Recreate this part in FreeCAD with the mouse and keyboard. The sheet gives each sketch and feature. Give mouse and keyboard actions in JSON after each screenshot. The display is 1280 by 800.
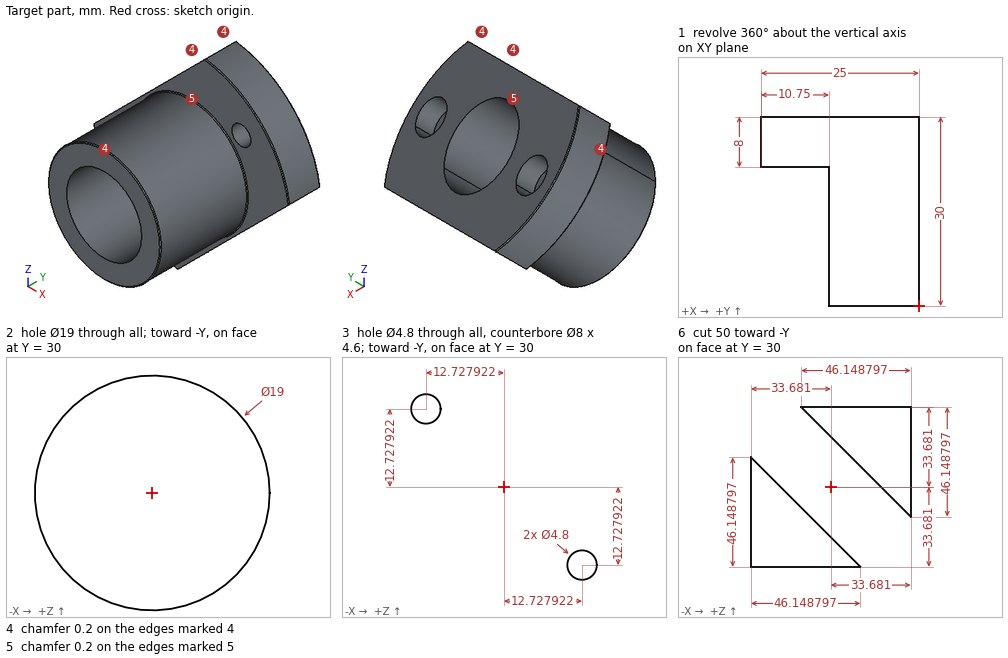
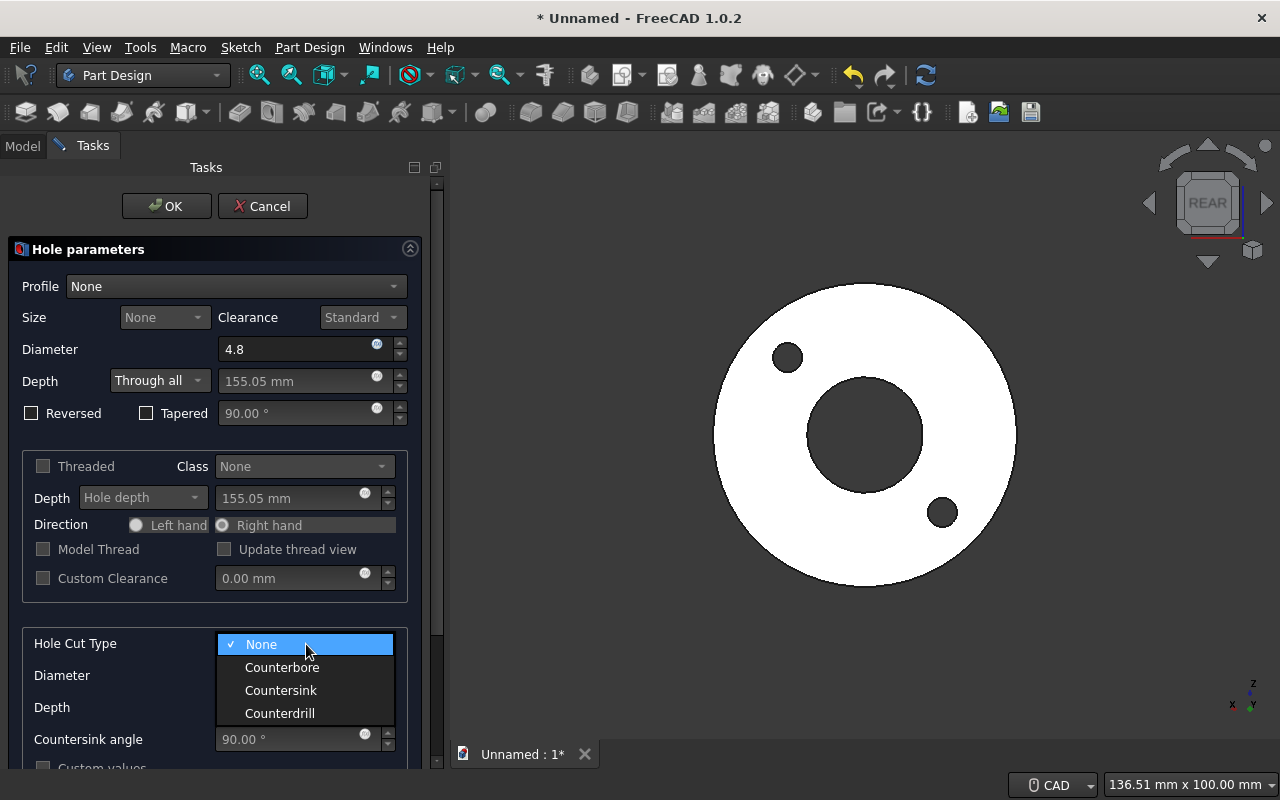
{"action": "left_click", "coordinate": [304, 668]}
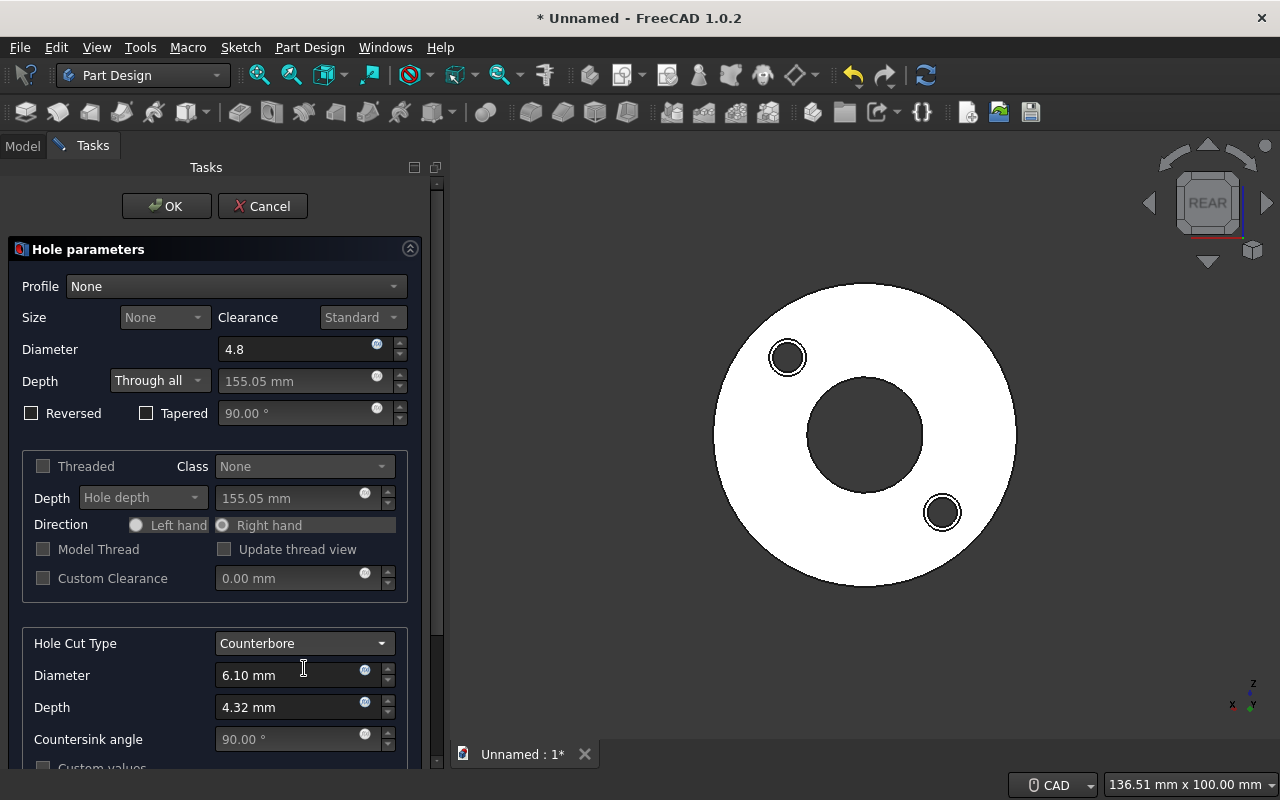
{"action": "triple_click", "coordinate": [298, 675]}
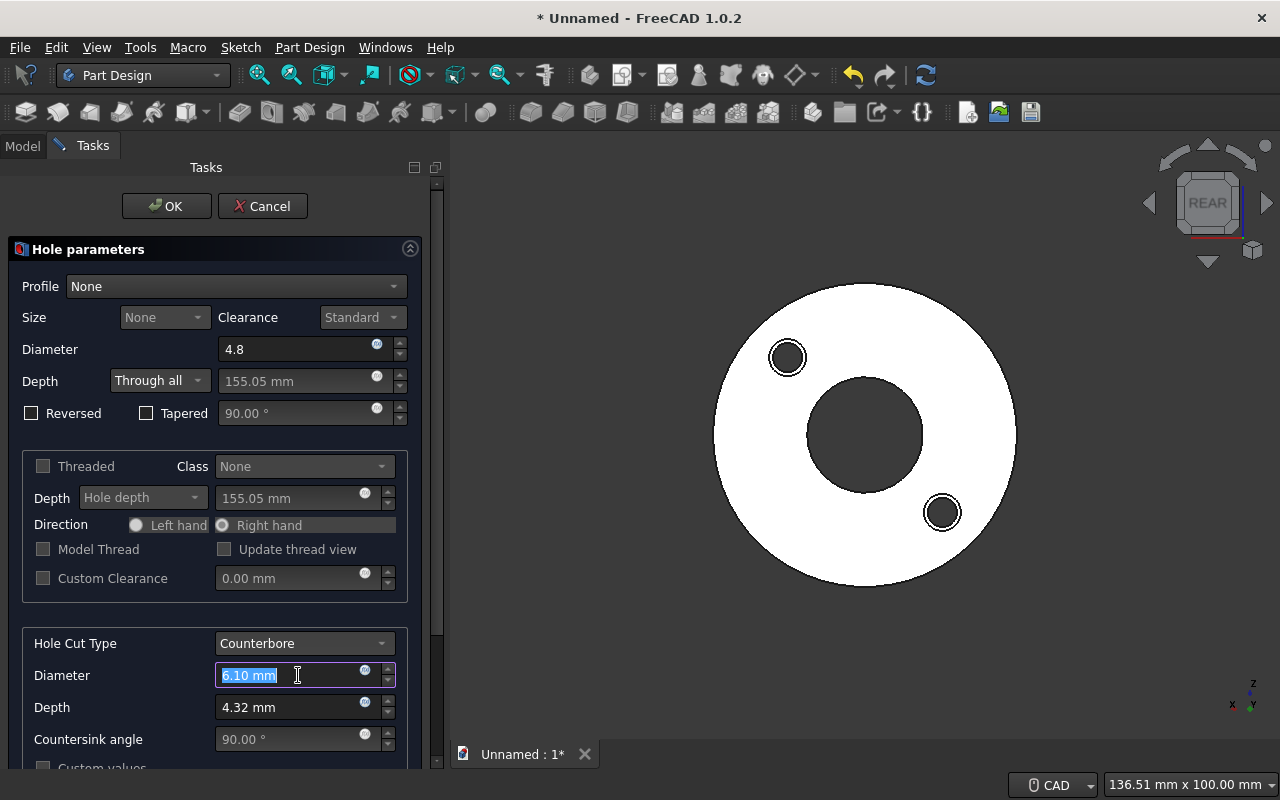
{"action": "type", "text": "8"}
{"action": "key", "text": "Tab"}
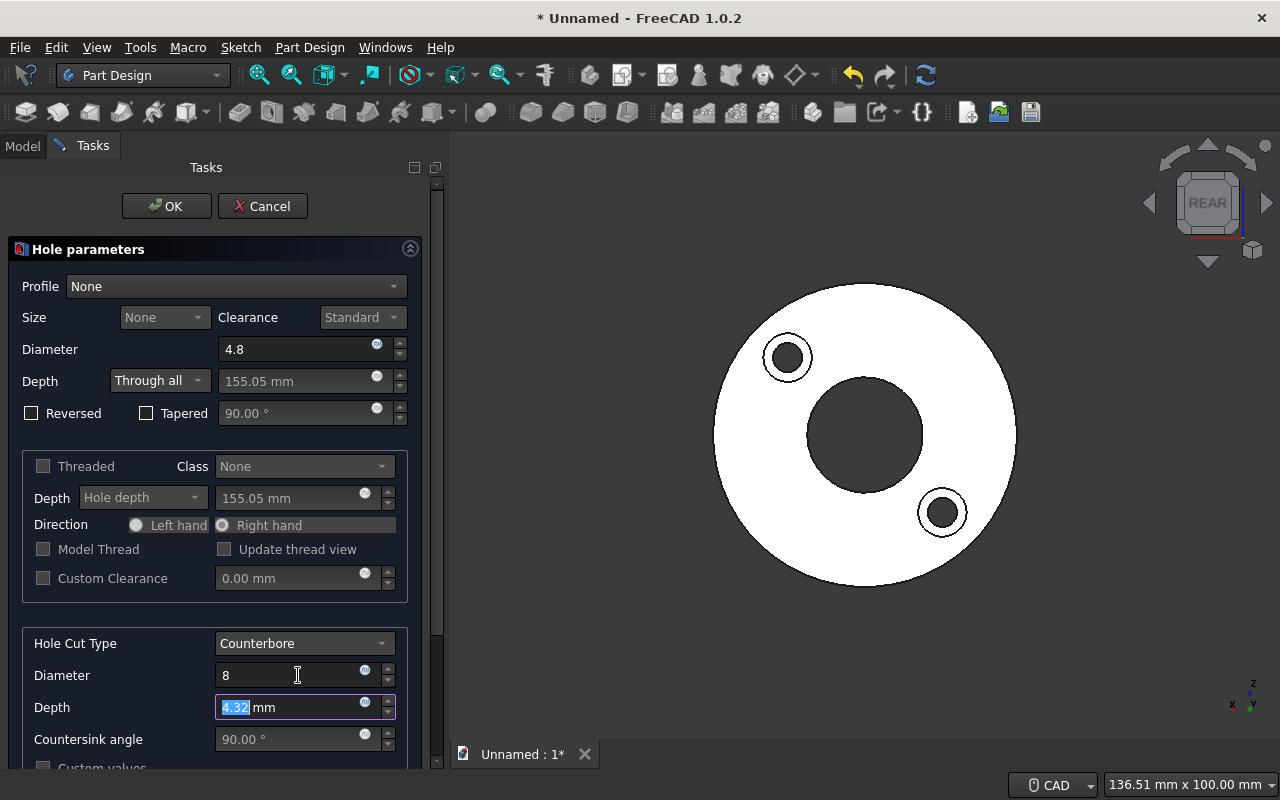
{"action": "type", "text": "4.6"}
{"action": "key", "text": "Tab"}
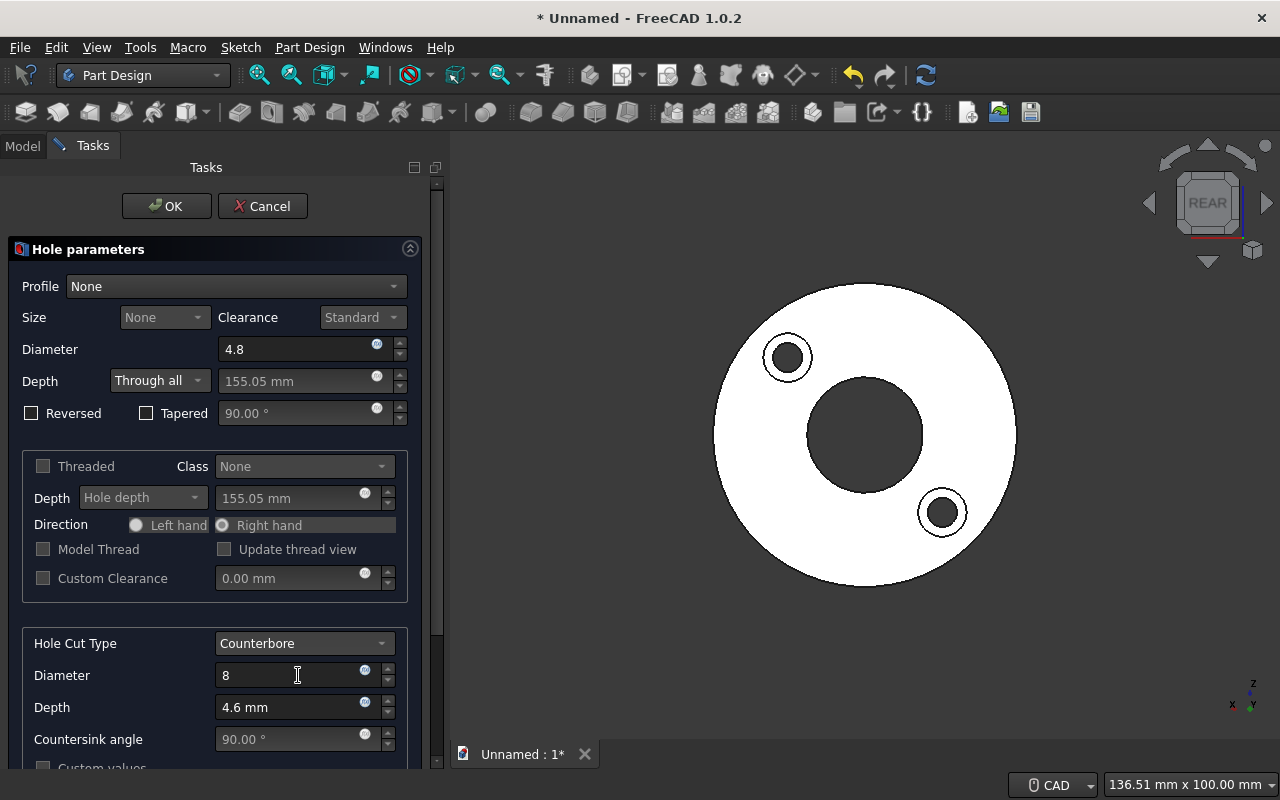
{"action": "left_click", "coordinate": [167, 206]}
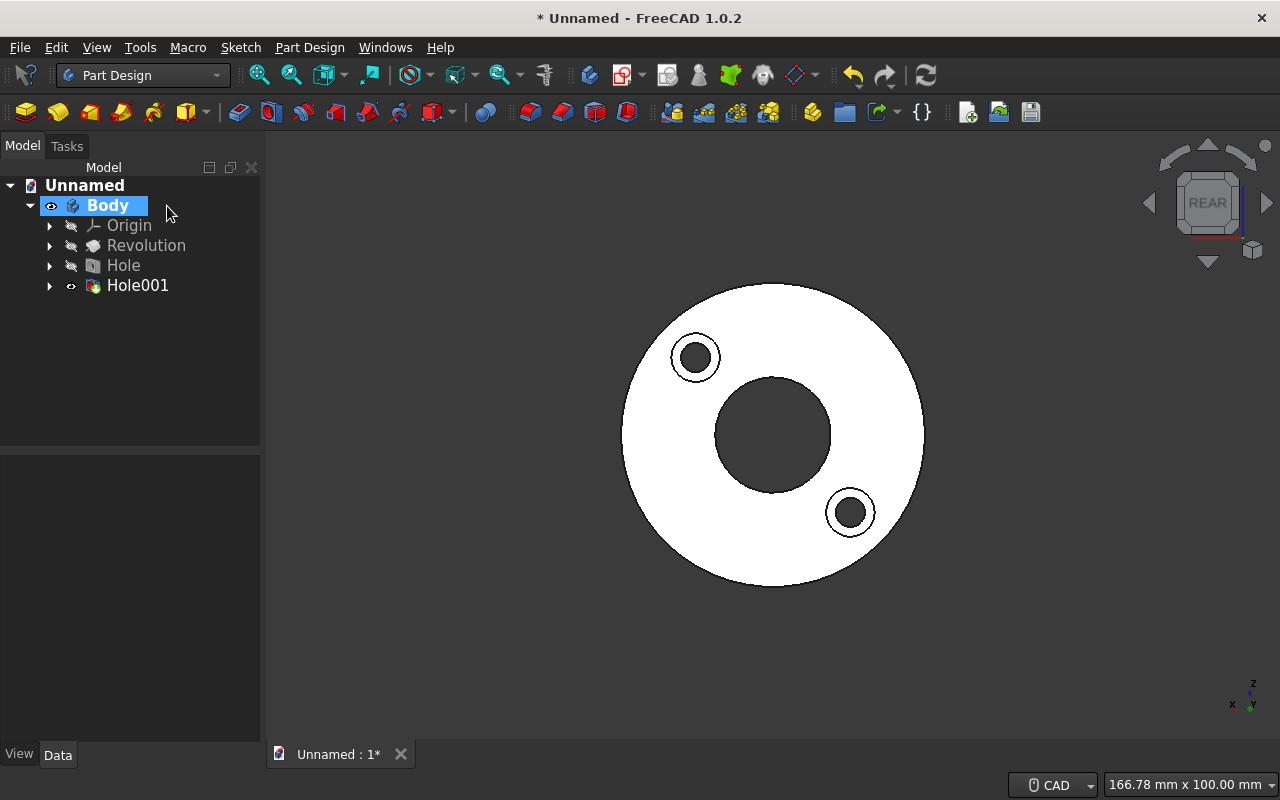
{"action": "left_click", "coordinate": [726, 289]}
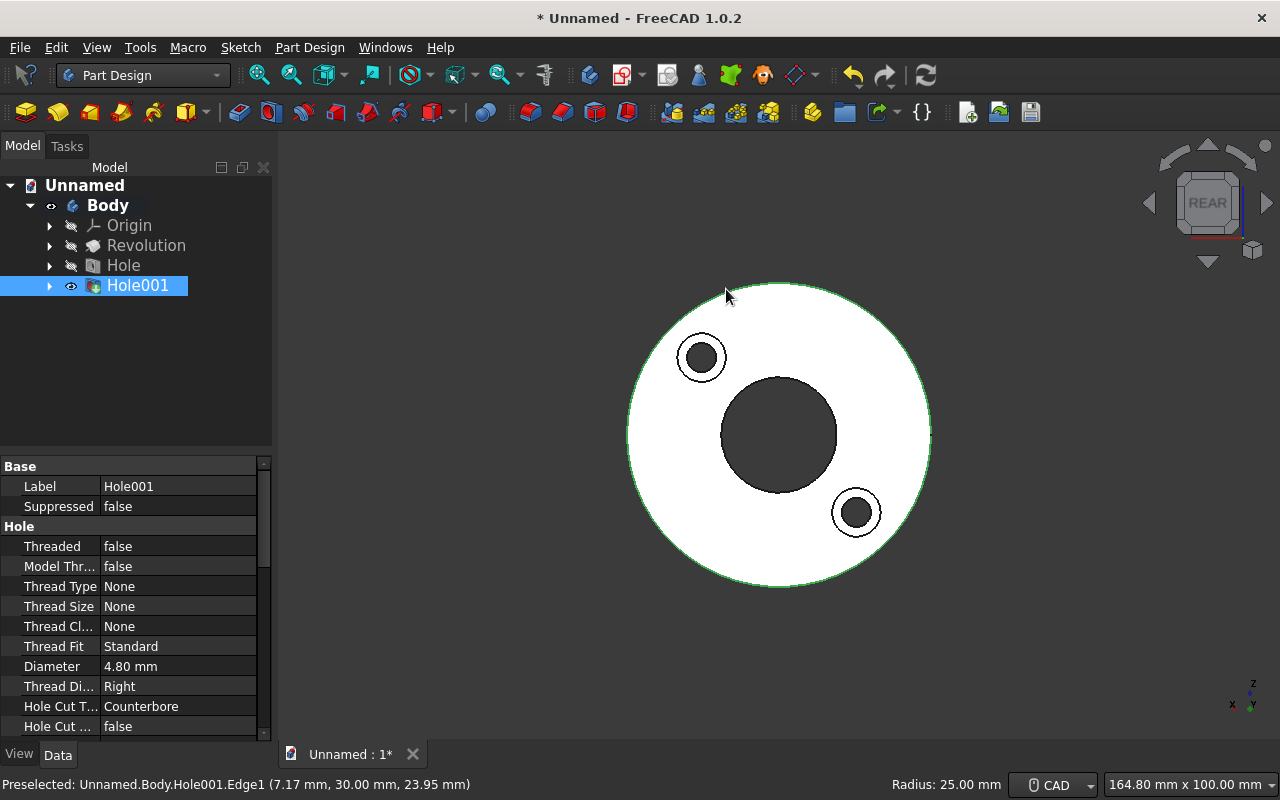
{"action": "key", "text": "0"}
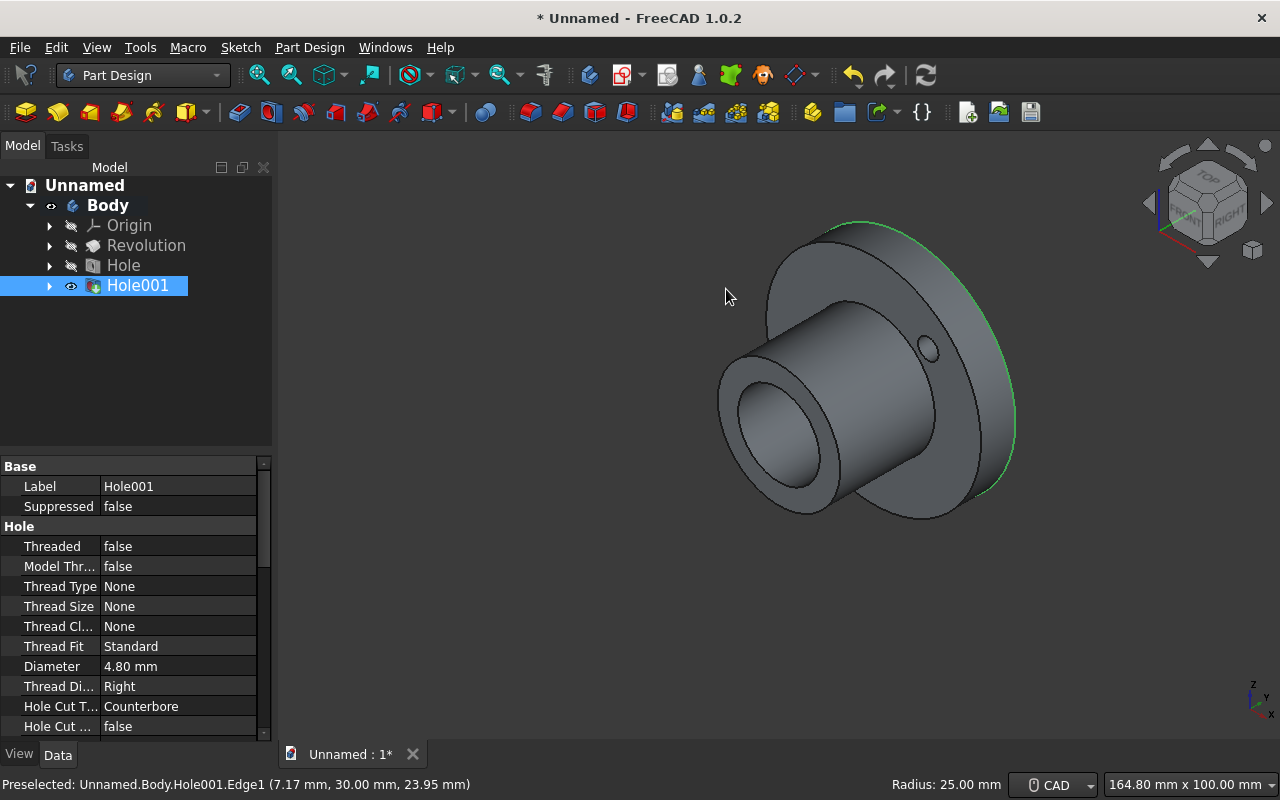
{"action": "left_click", "coordinate": [840, 469], "text": "ctrl"}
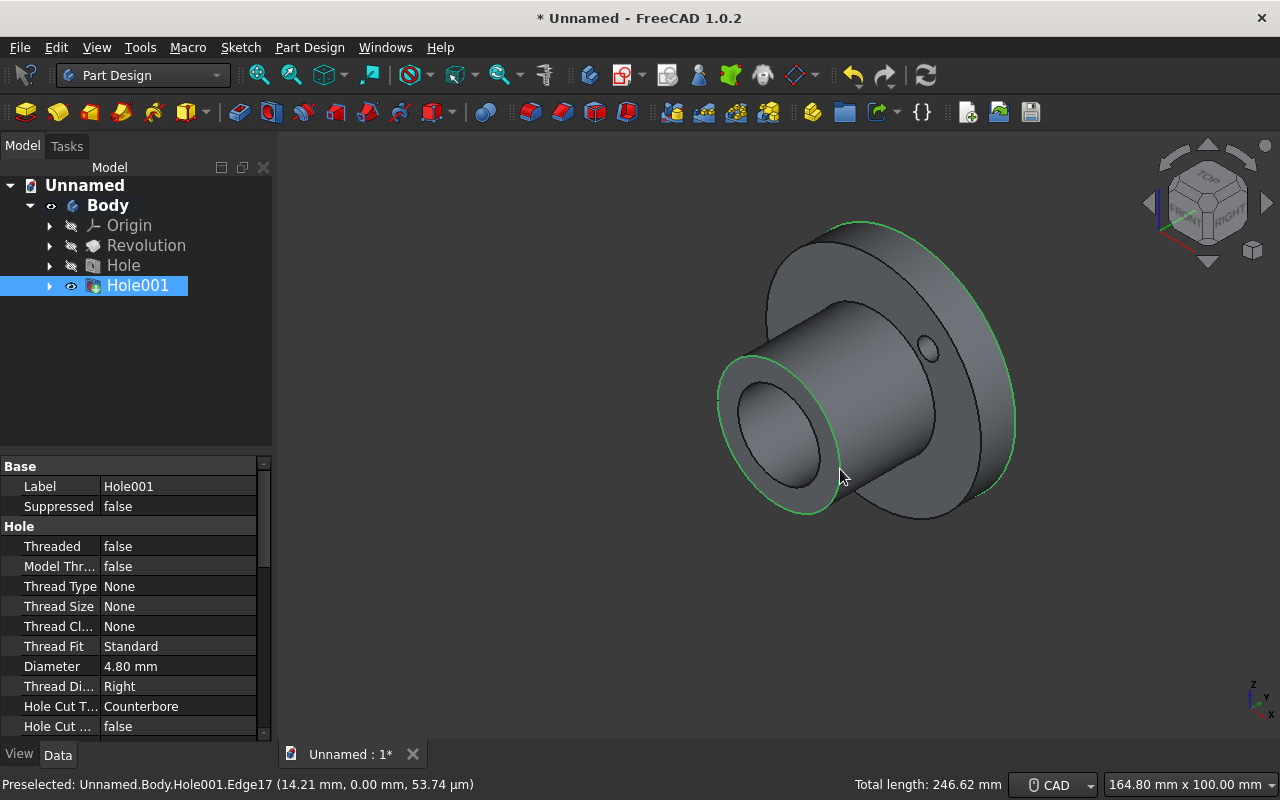
{"action": "left_click", "coordinate": [981, 441], "text": "ctrl"}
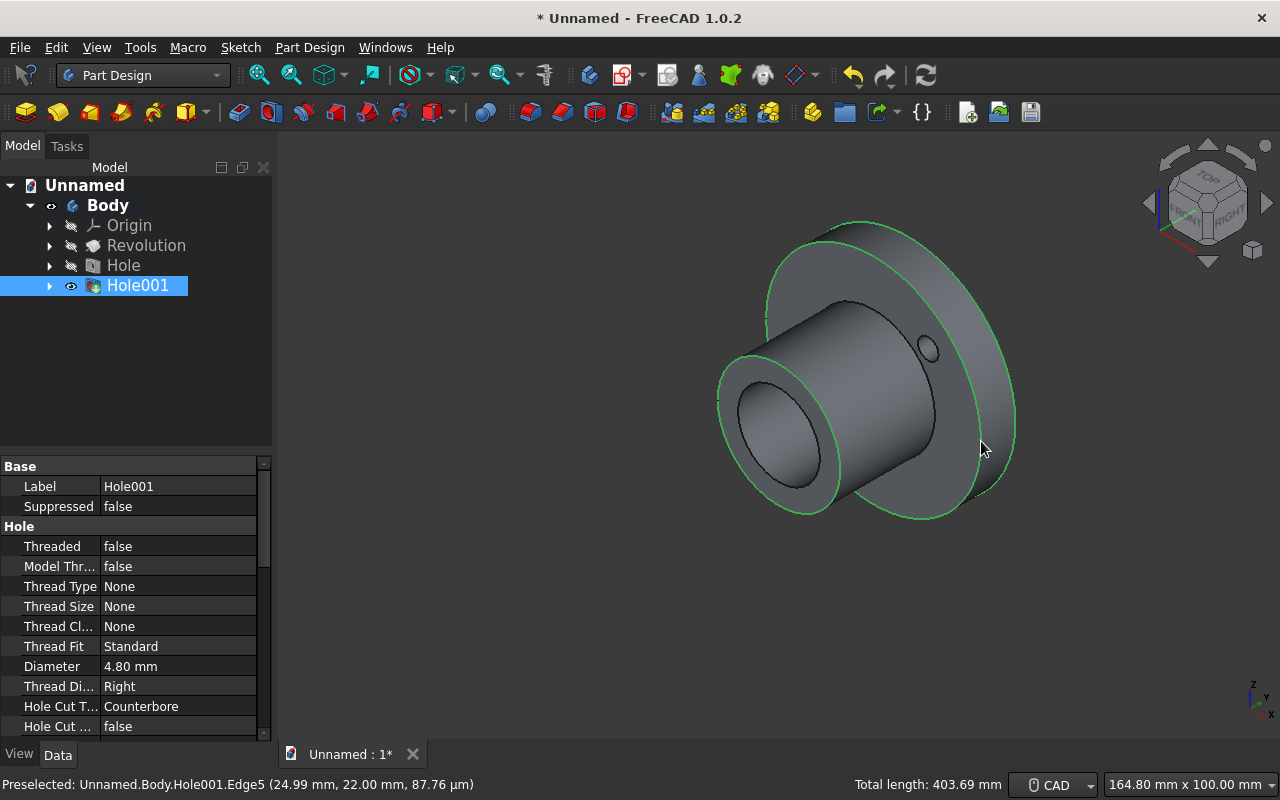
{"action": "left_click", "coordinate": [564, 112]}